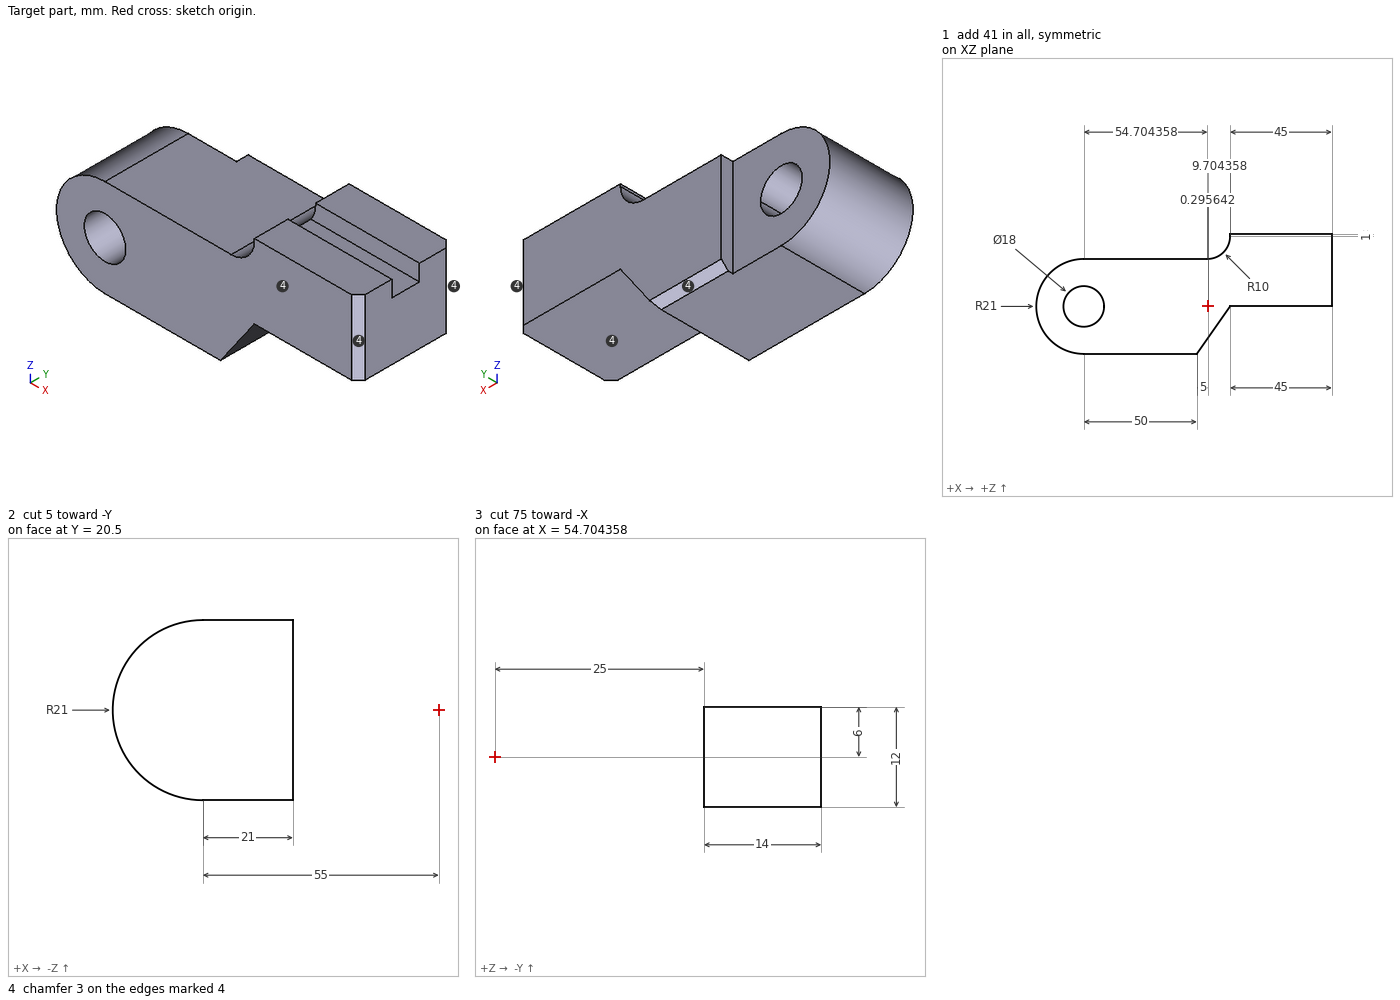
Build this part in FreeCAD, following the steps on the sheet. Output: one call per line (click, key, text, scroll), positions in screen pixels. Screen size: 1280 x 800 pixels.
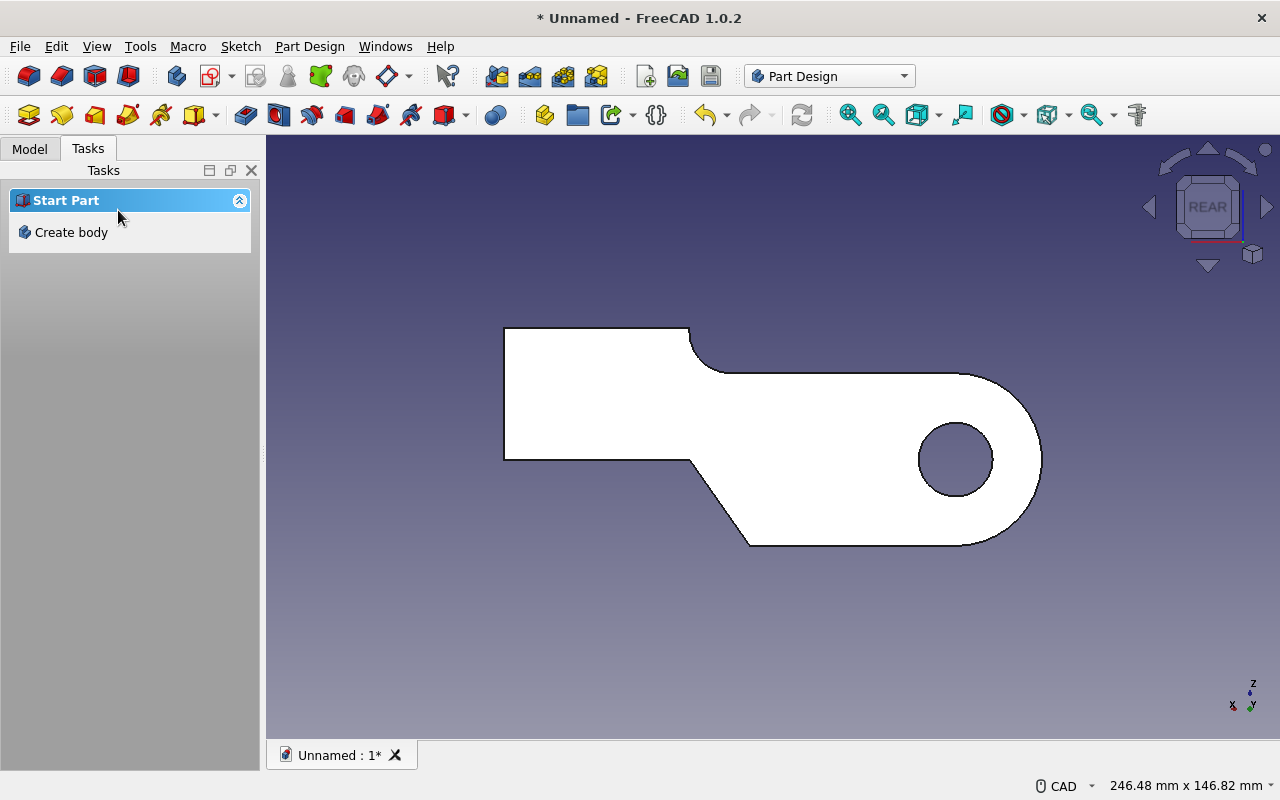
click(850, 467)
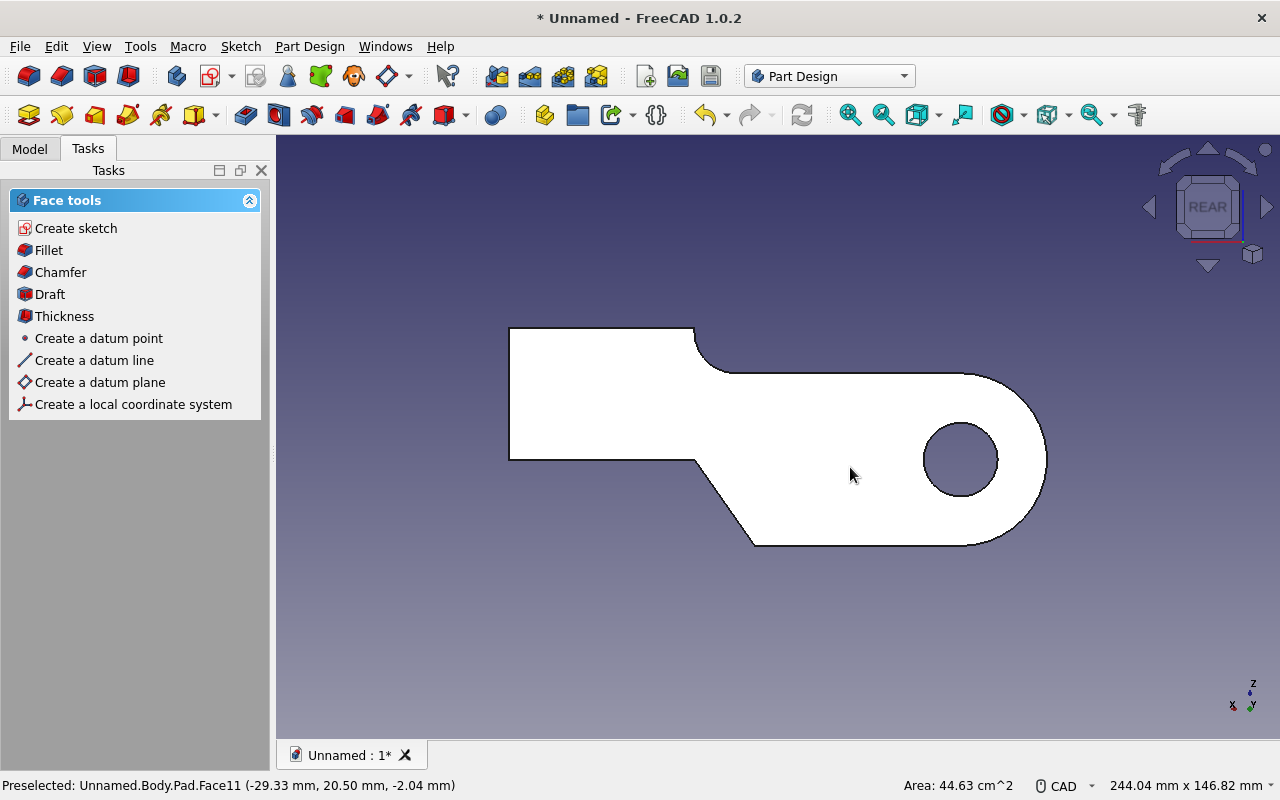
click(210, 76)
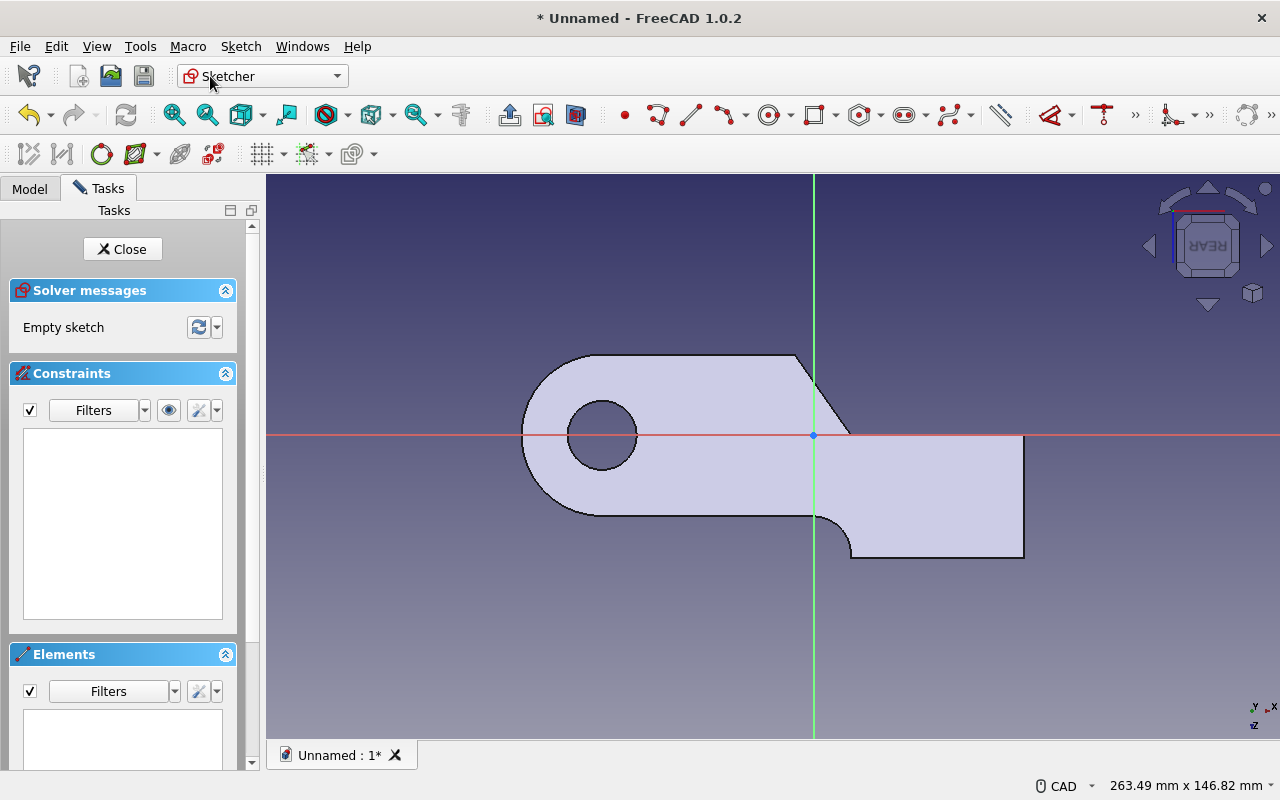
scroll(623, 410, up, 3)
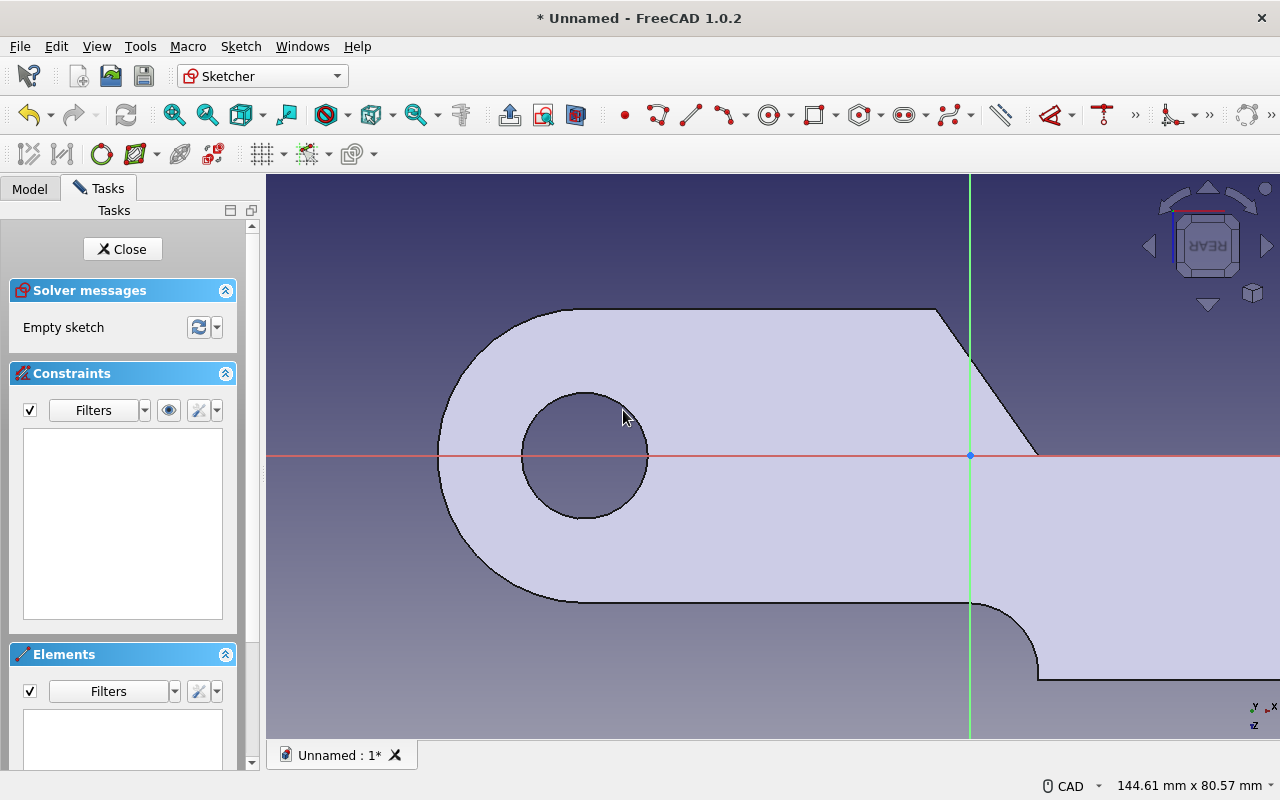
click(658, 116)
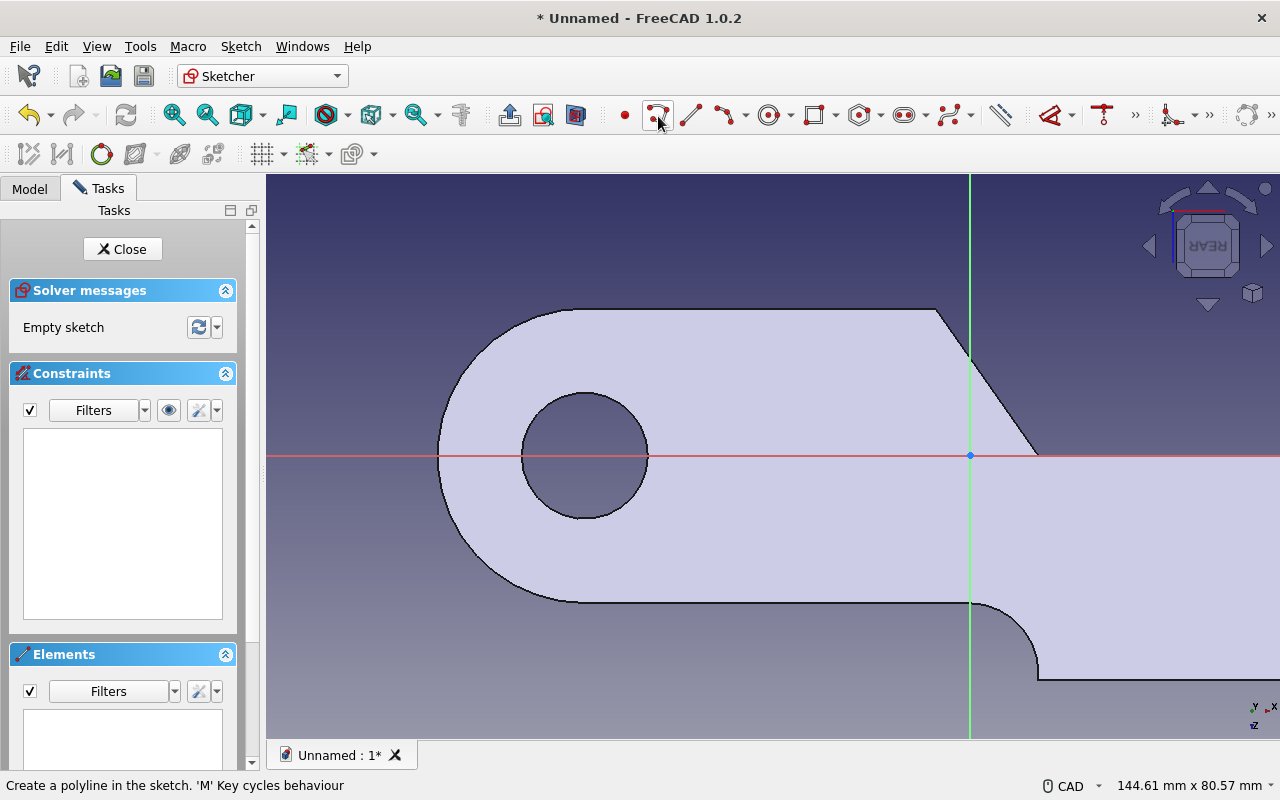
click(585, 603)
click(732, 603)
click(732, 309)
click(585, 309)
right_click(585, 309)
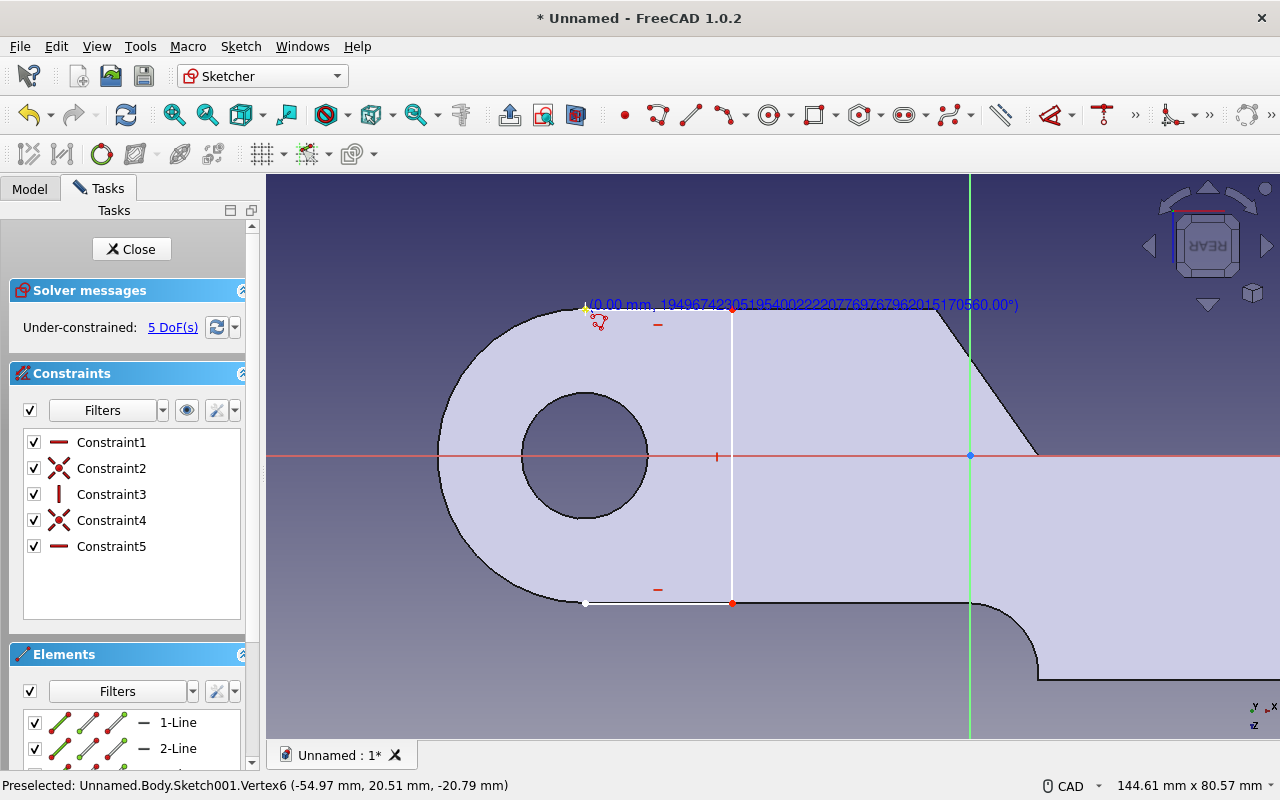
click(724, 116)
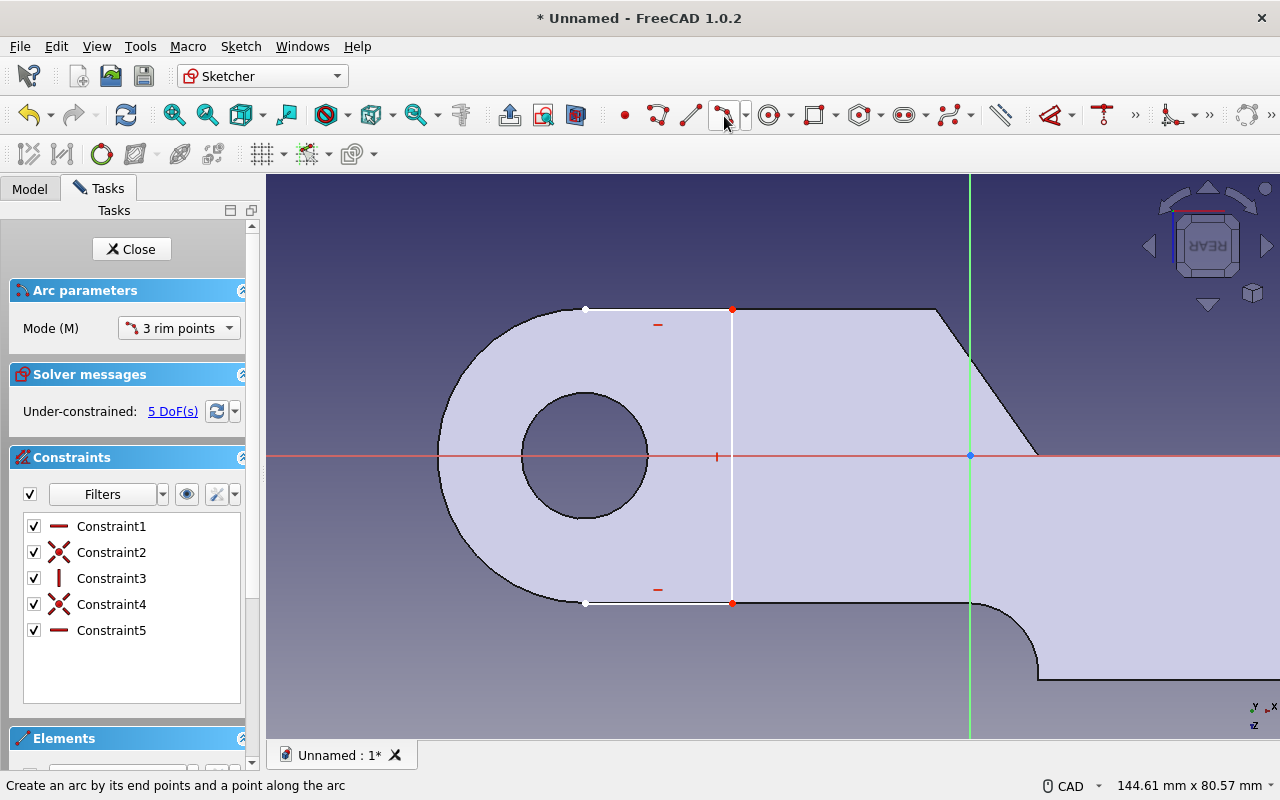
click(585, 310)
click(585, 604)
click(445, 410)
key(Escape)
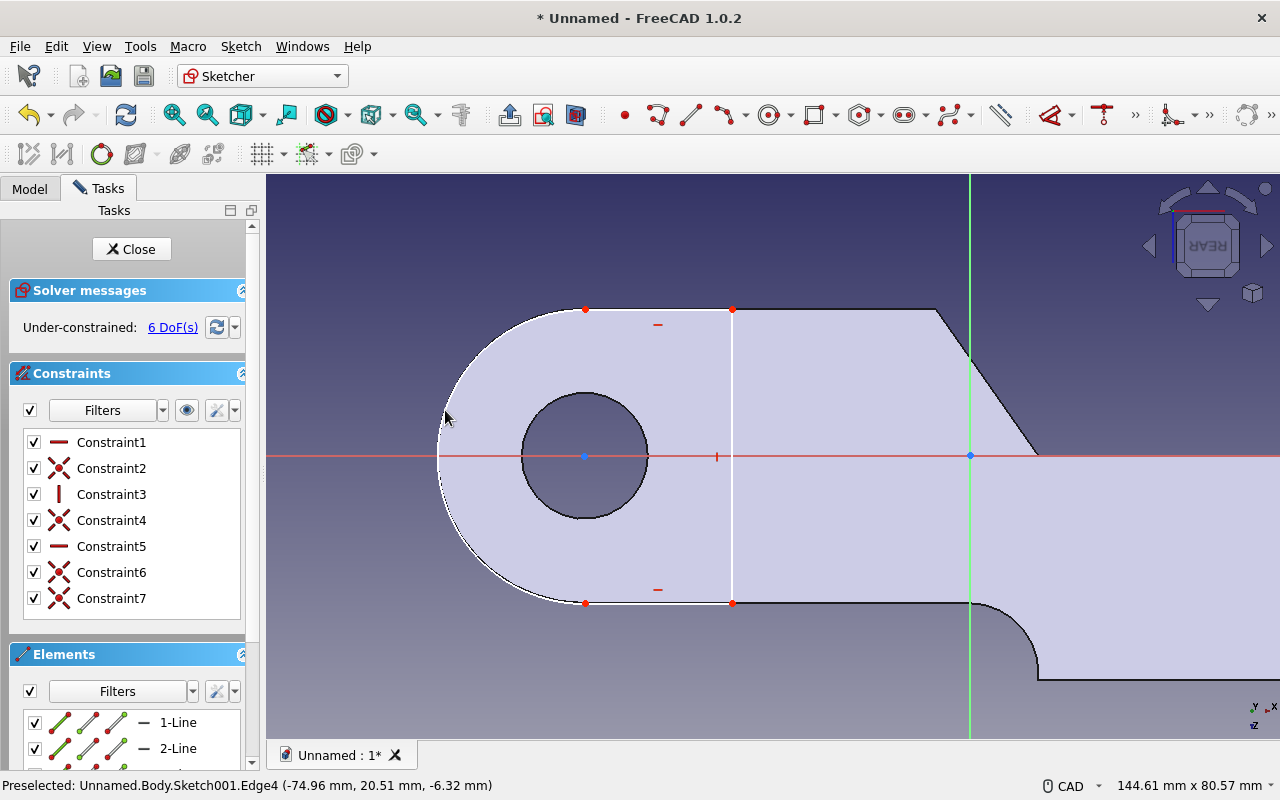
click(629, 604)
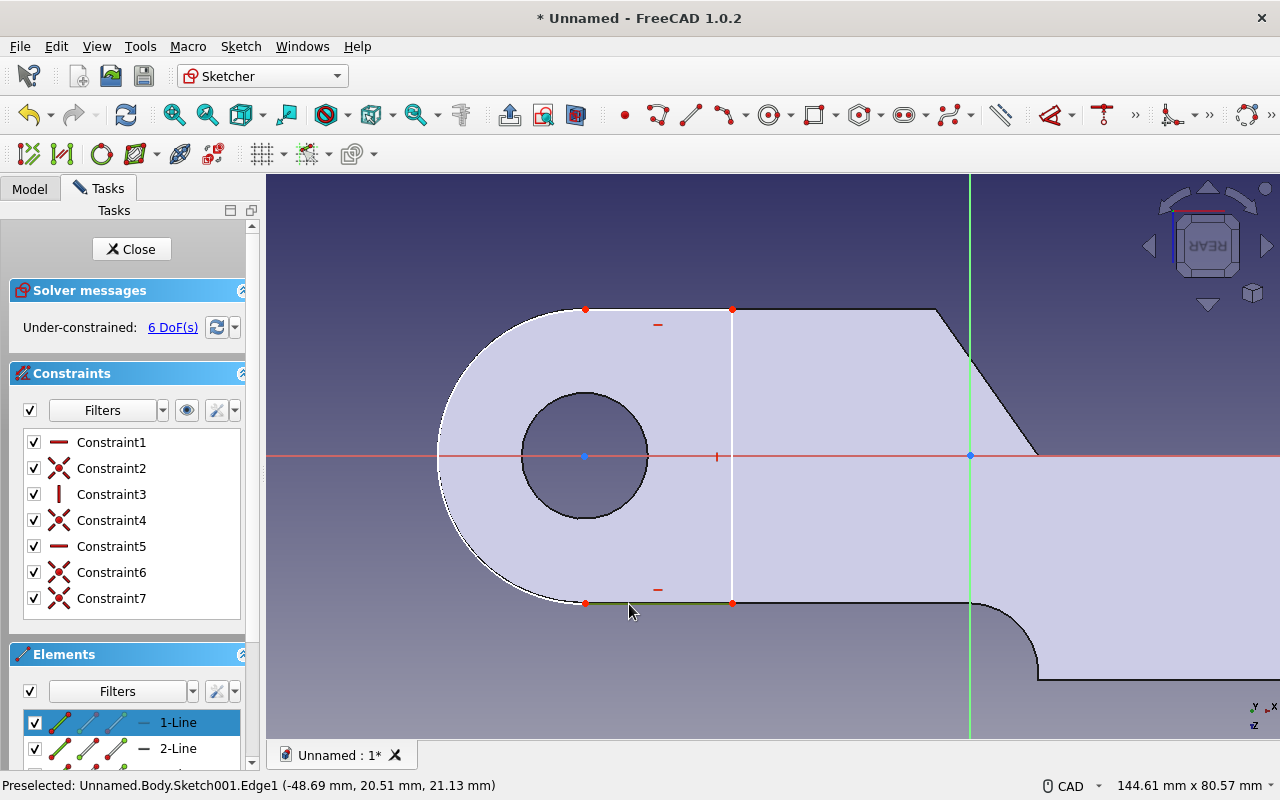
click(466, 370)